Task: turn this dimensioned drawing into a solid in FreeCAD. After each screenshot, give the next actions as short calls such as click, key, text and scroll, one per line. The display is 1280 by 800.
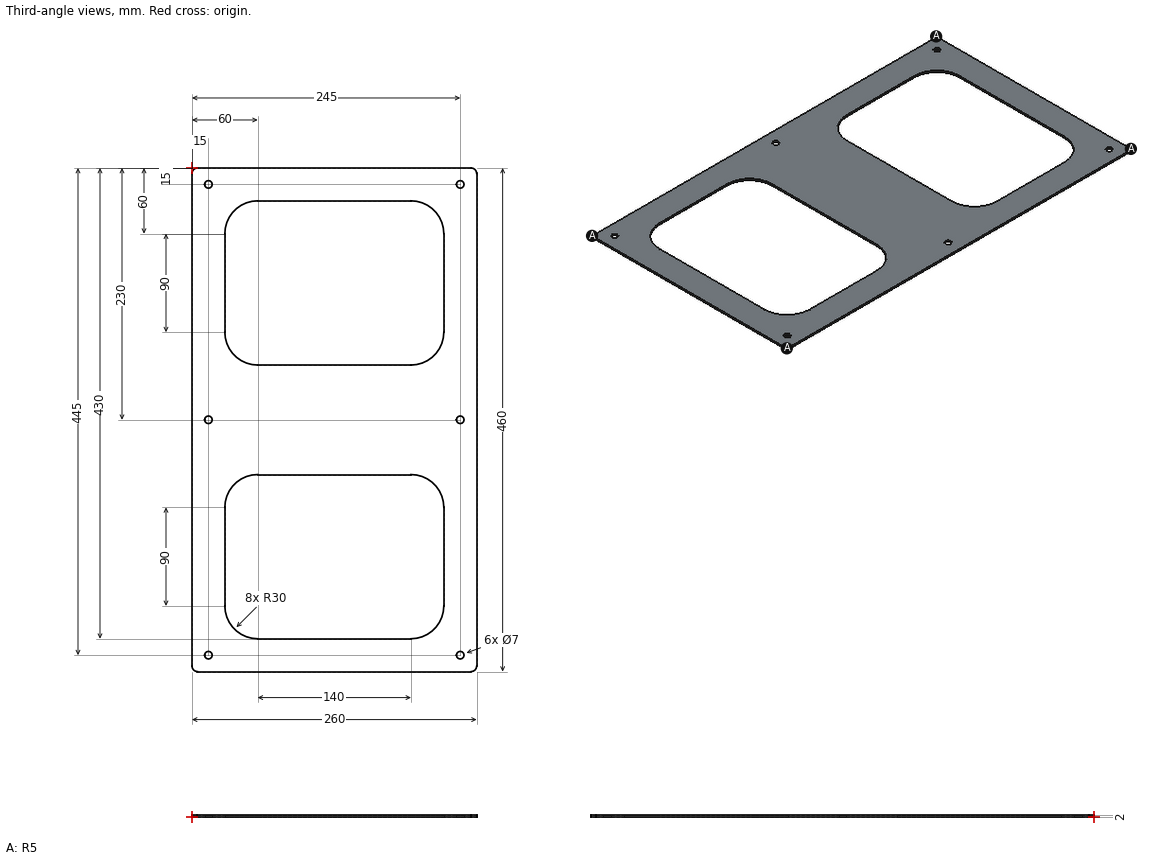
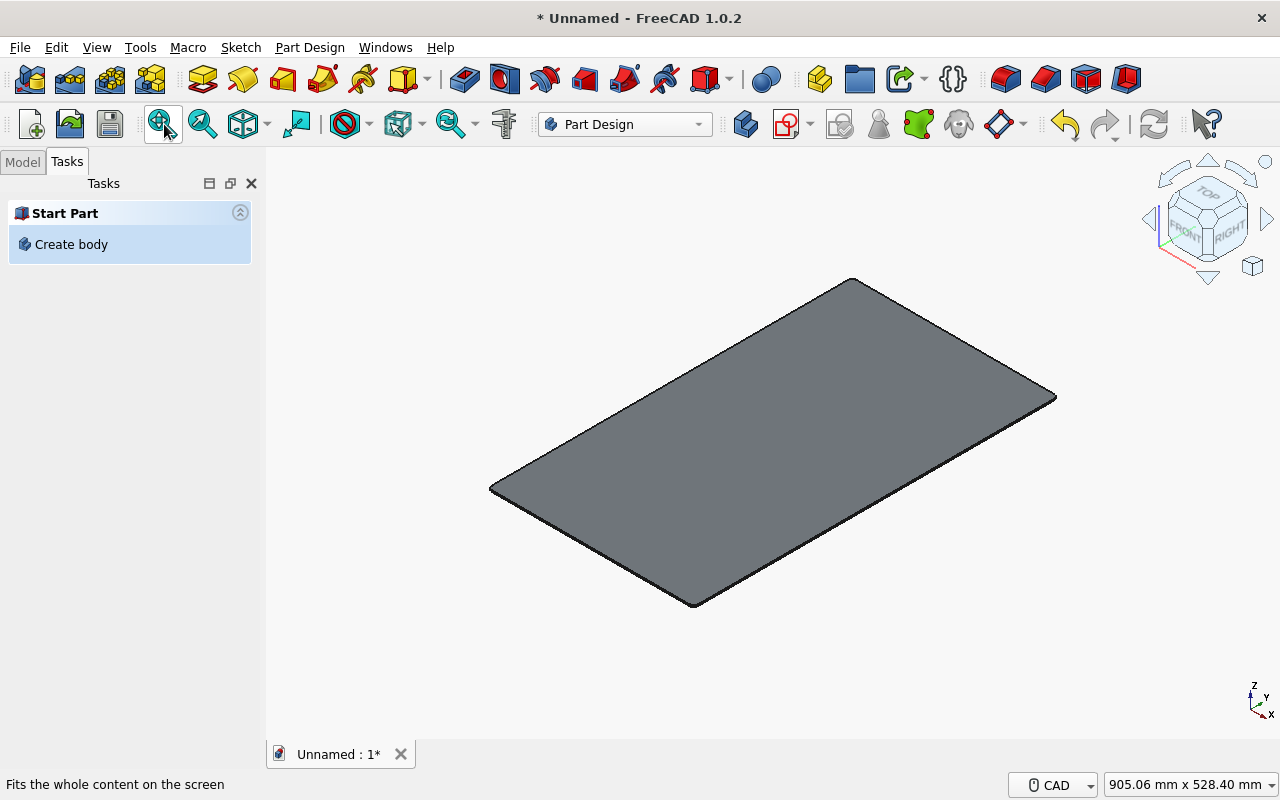
click(786, 124)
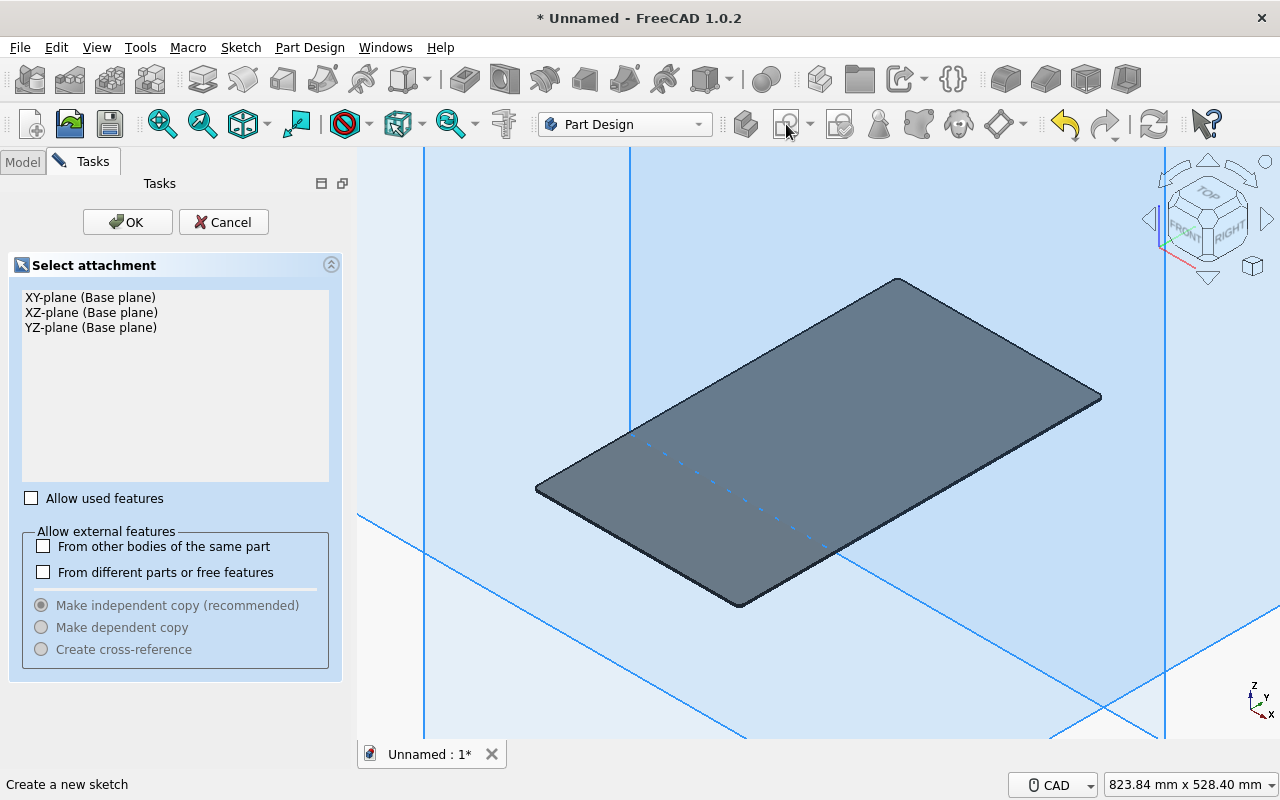
click(82, 298)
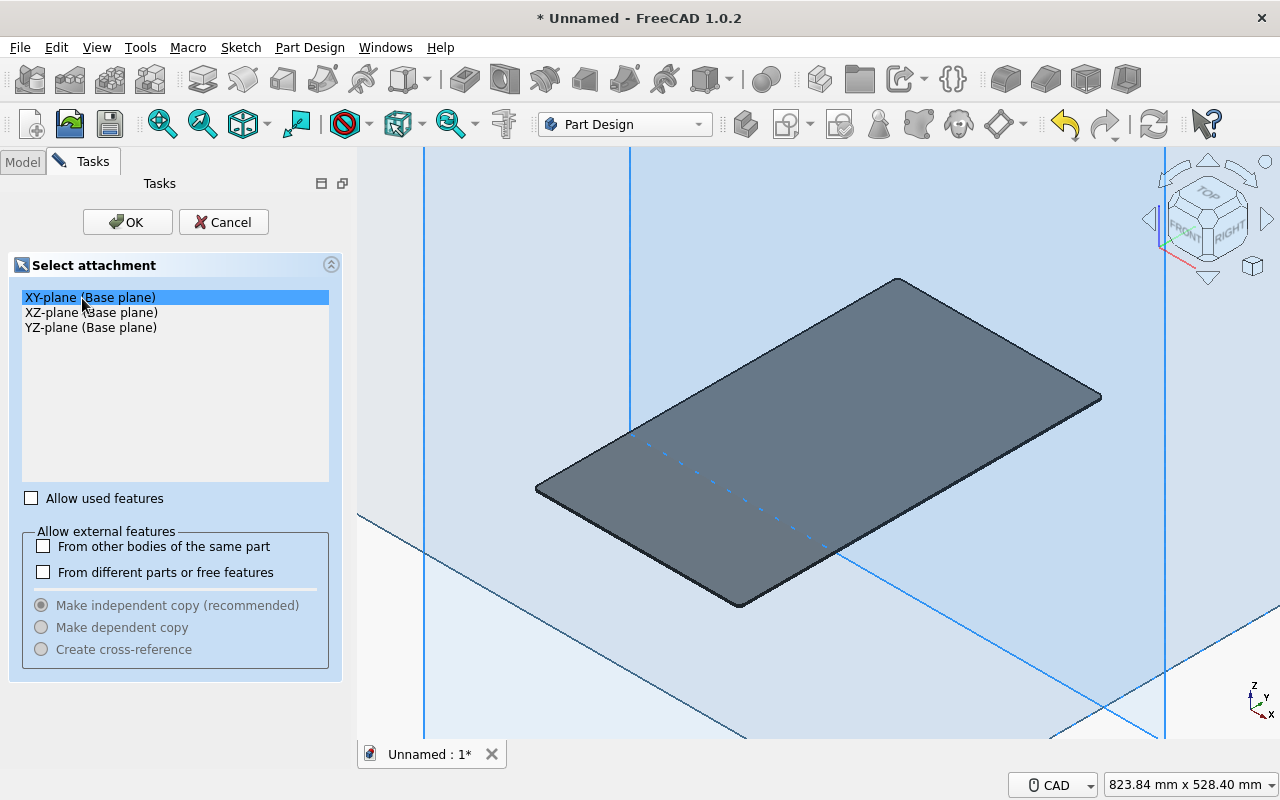
click(128, 222)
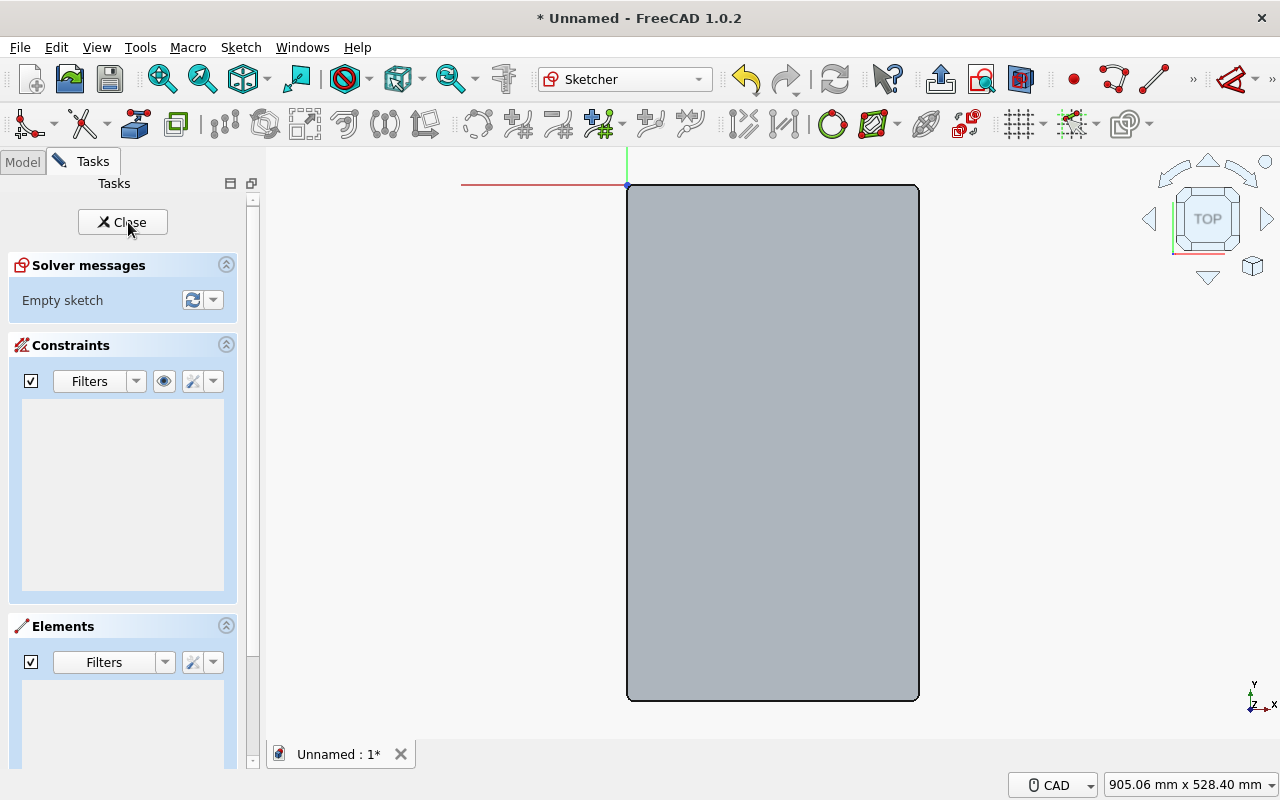
click(1022, 80)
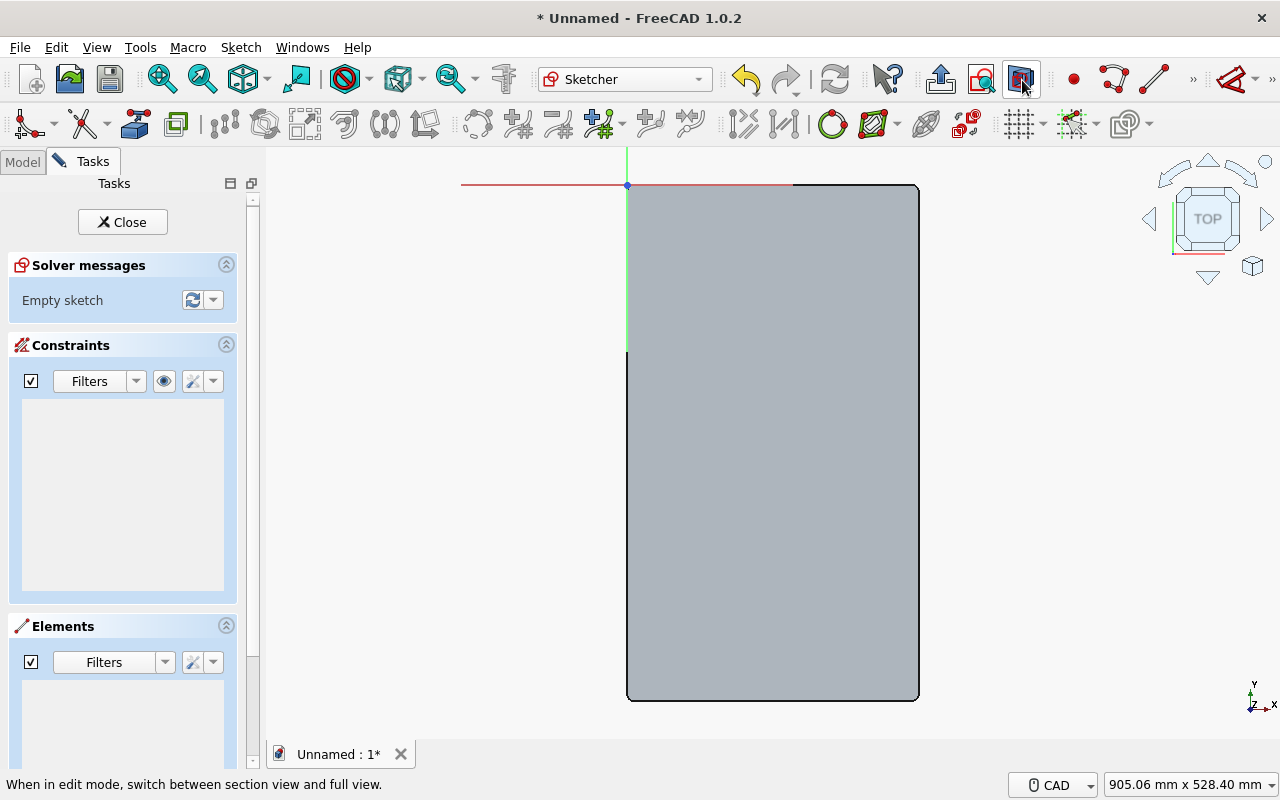
scroll(424, 472, down, 1)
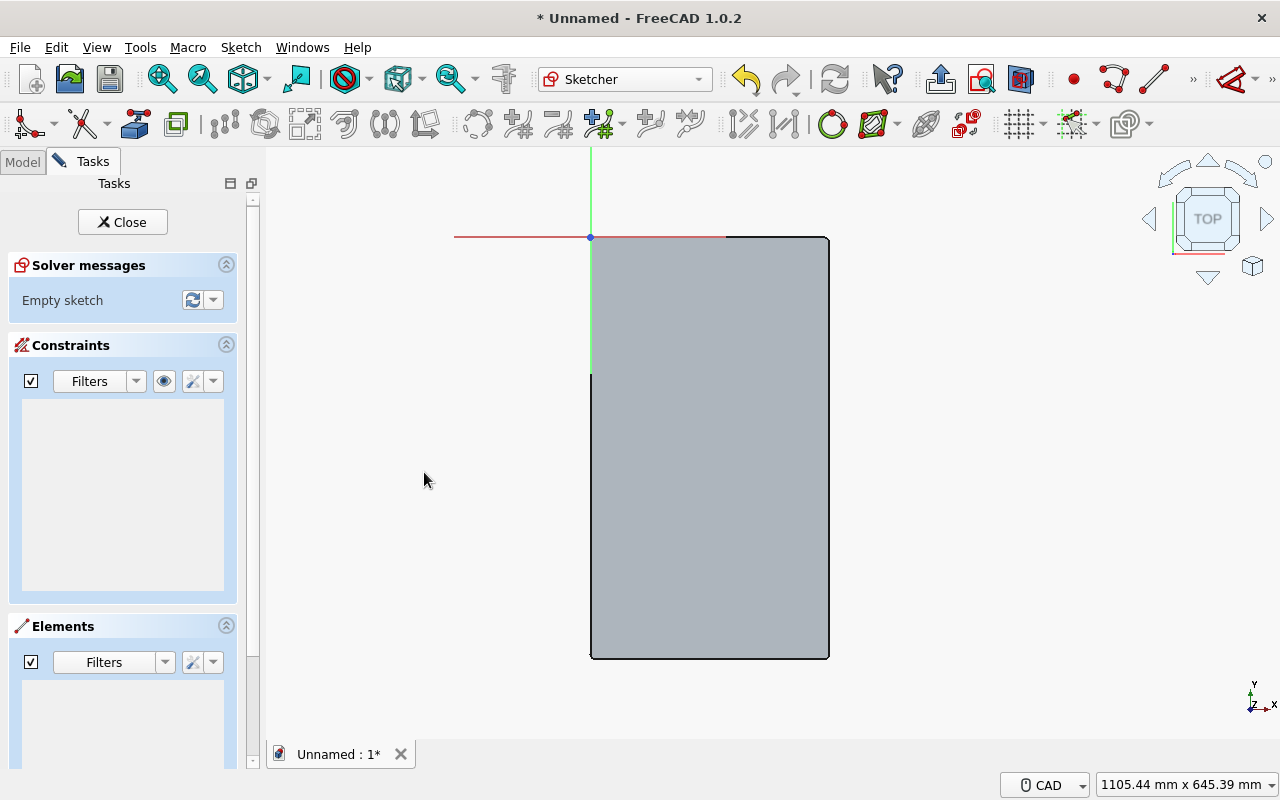
key(g)
key(c)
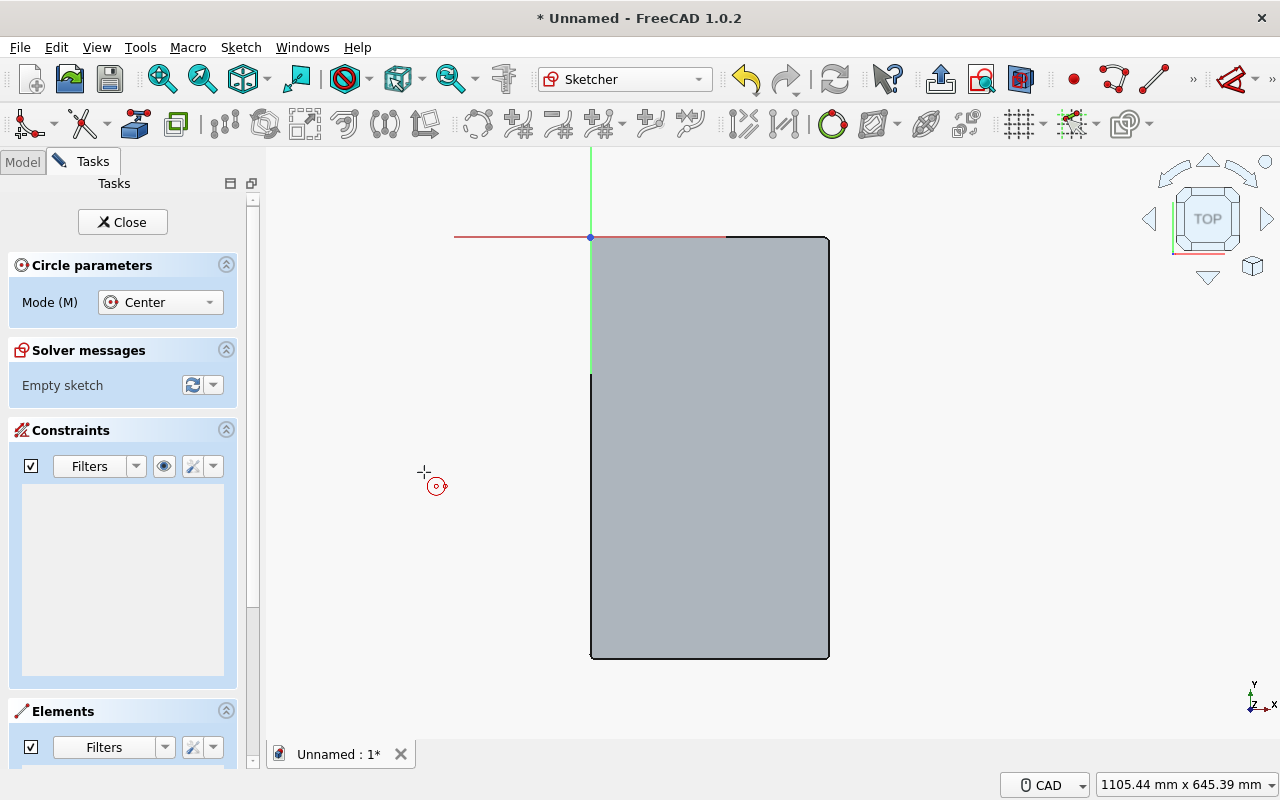
scroll(815, 646, up, 10)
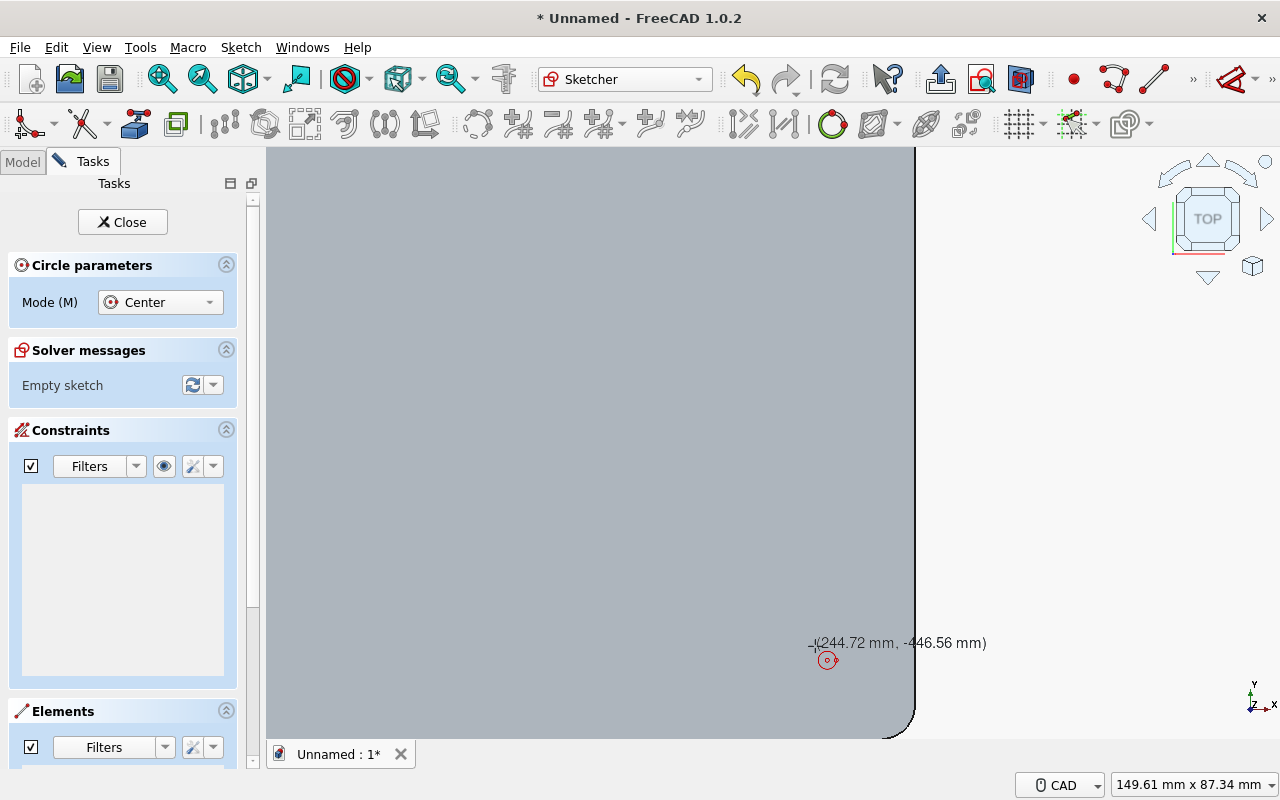
scroll(816, 647, down, 10)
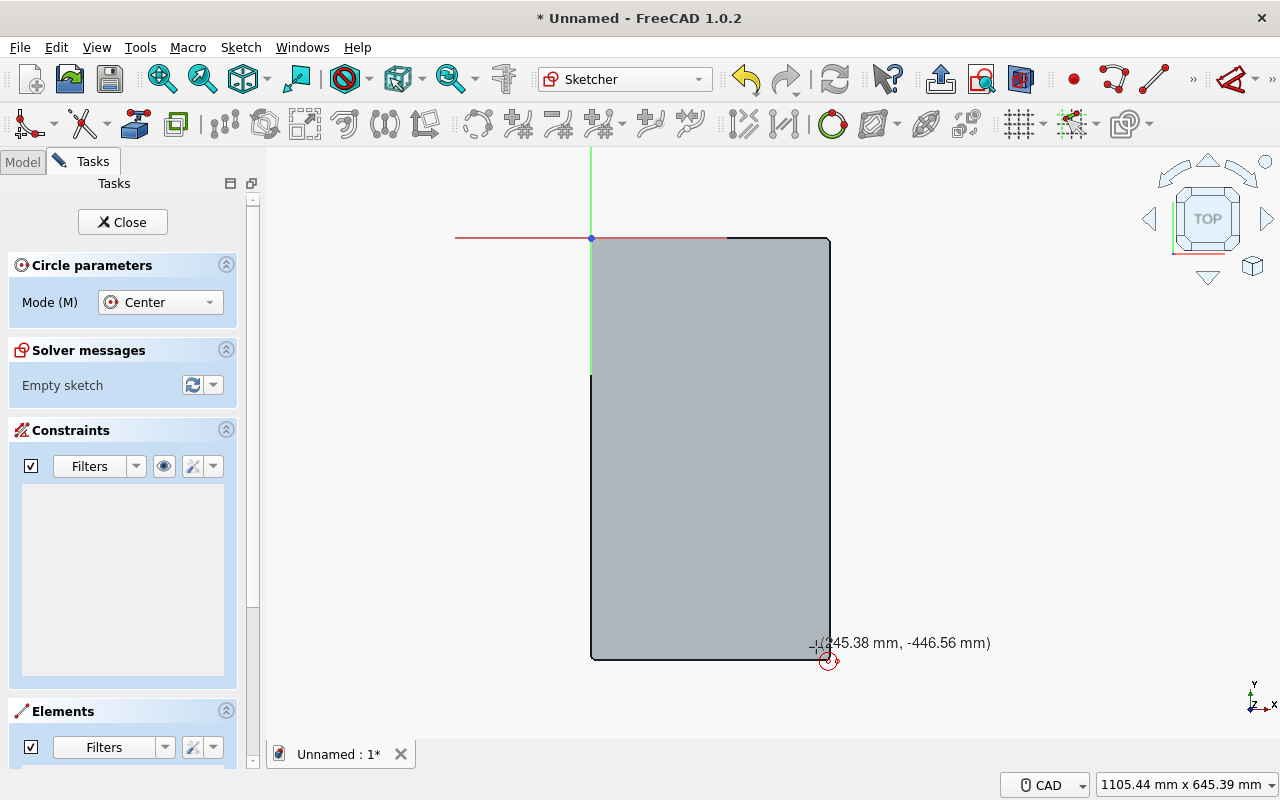
click(816, 646)
move(818, 644)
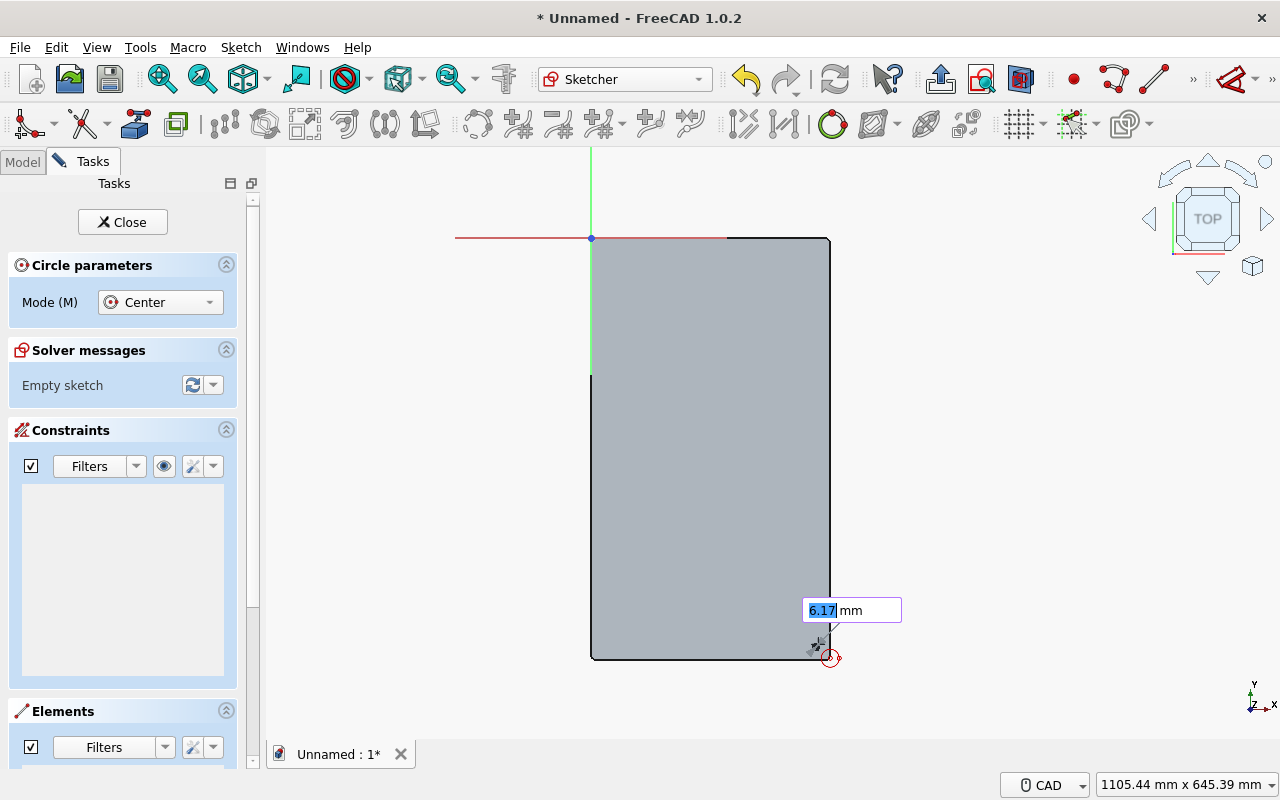
text(7)
key(Return)